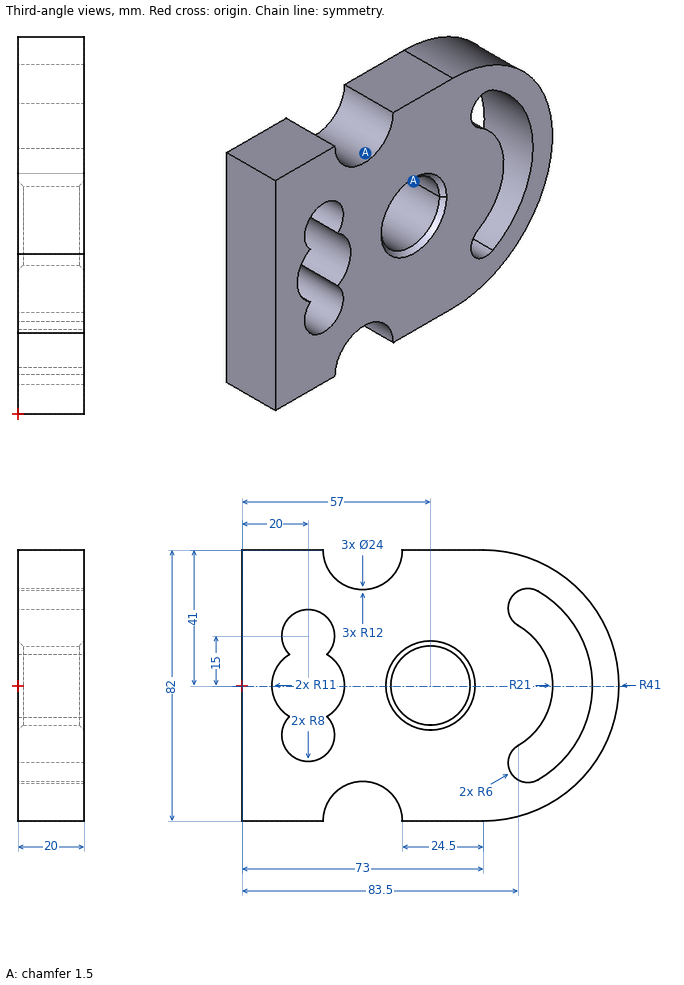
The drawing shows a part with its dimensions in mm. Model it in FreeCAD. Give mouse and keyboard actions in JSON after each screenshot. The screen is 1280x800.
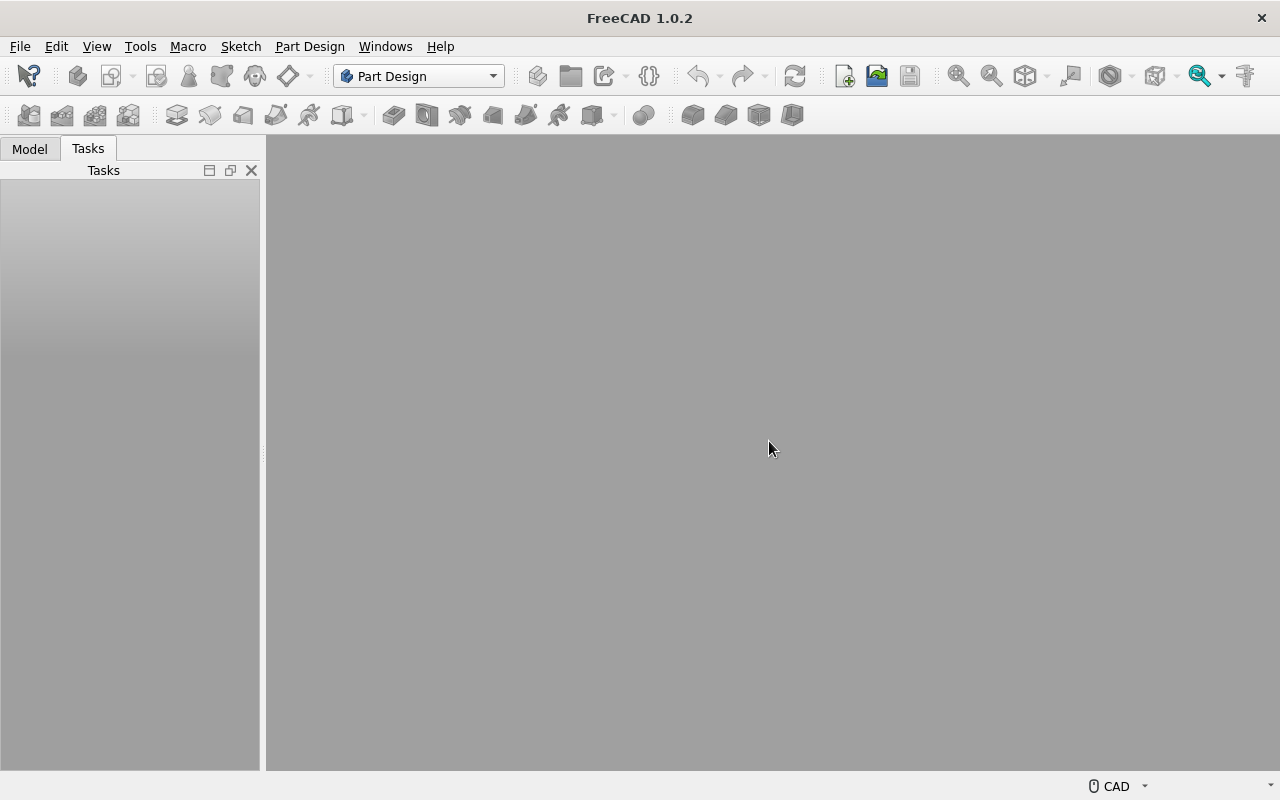
{"action": "key", "text": "ctrl+n"}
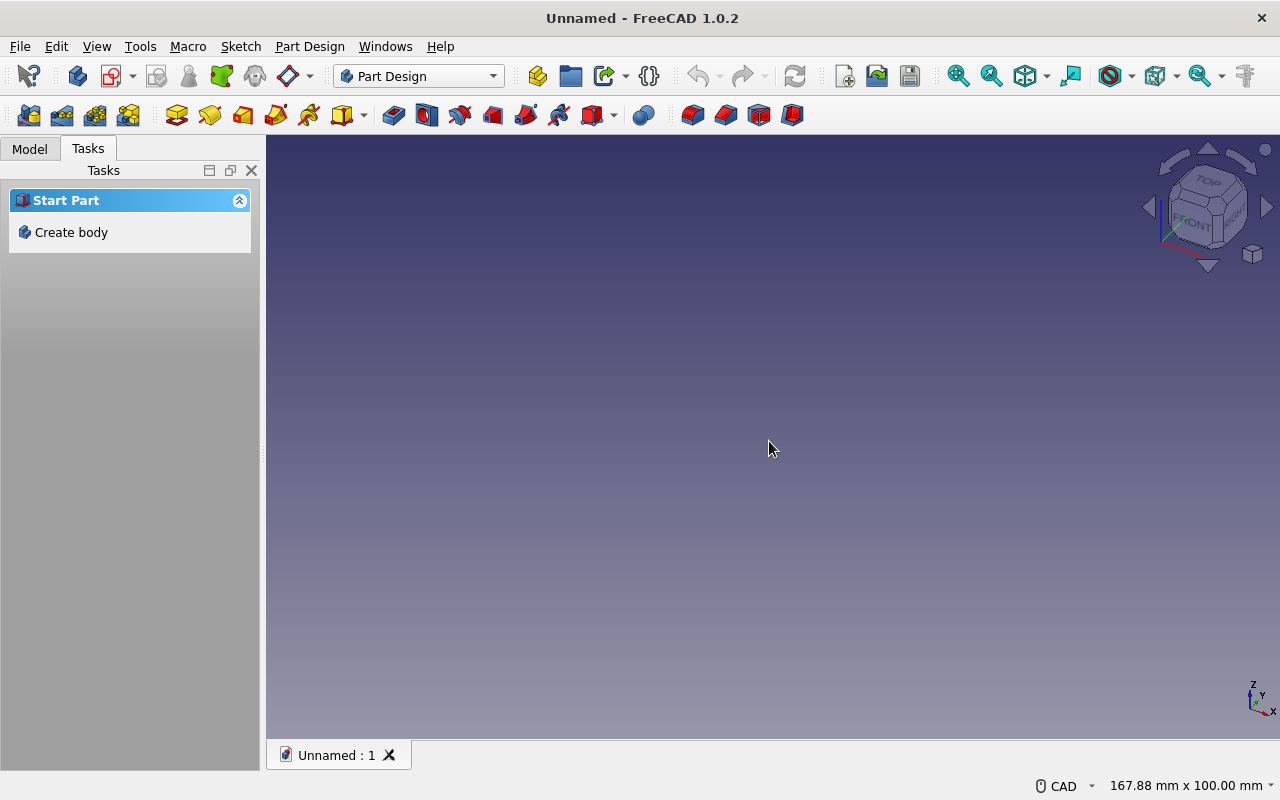
{"action": "left_click", "coordinate": [110, 76]}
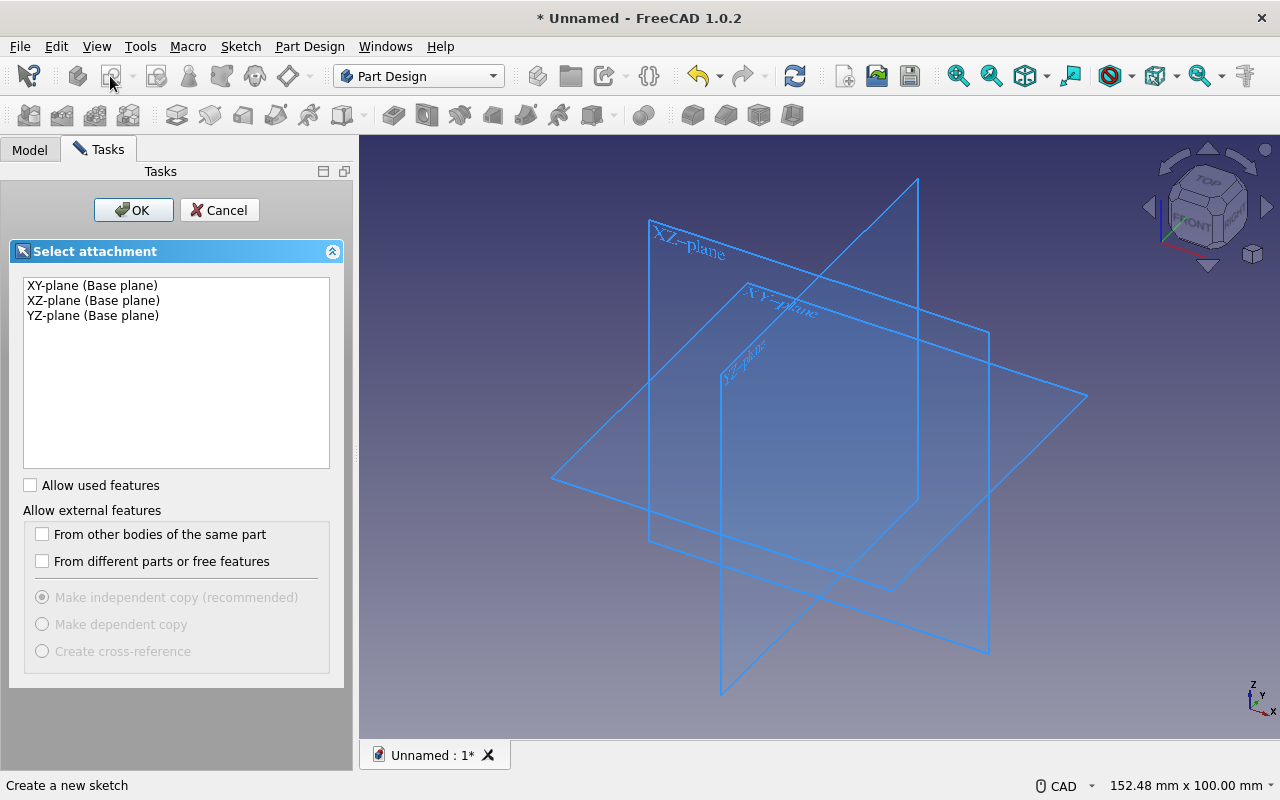
{"action": "left_click", "coordinate": [84, 316]}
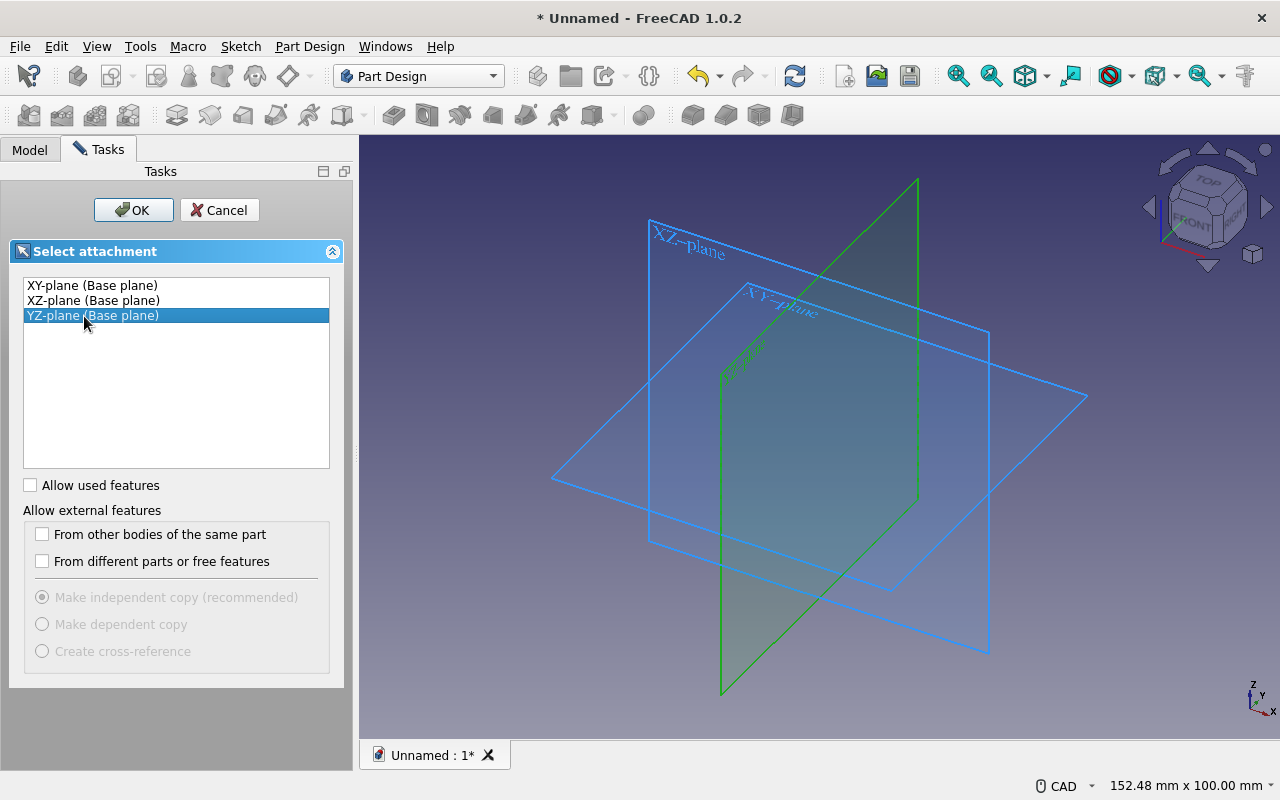
{"action": "left_click", "coordinate": [134, 210]}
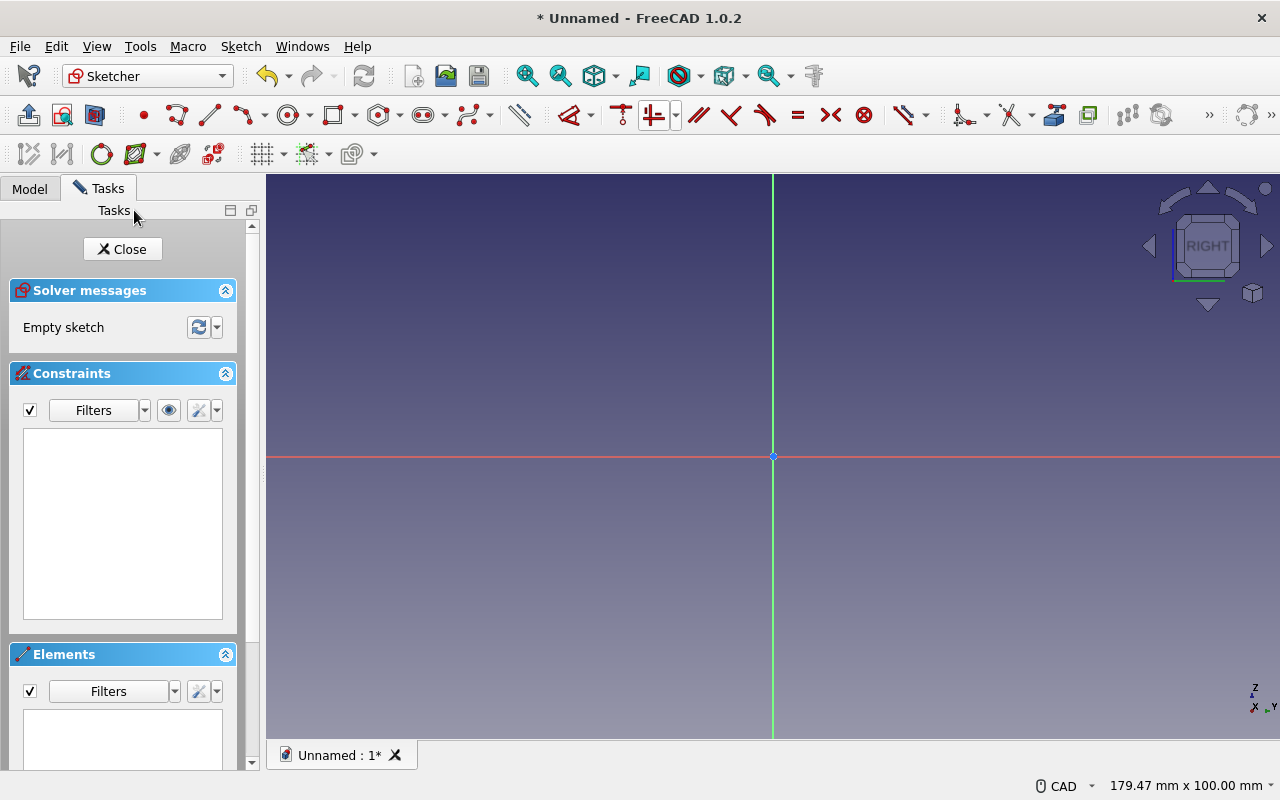
{"action": "scroll", "coordinate": [294, 457], "scroll_direction": "down", "scroll_amount": 2}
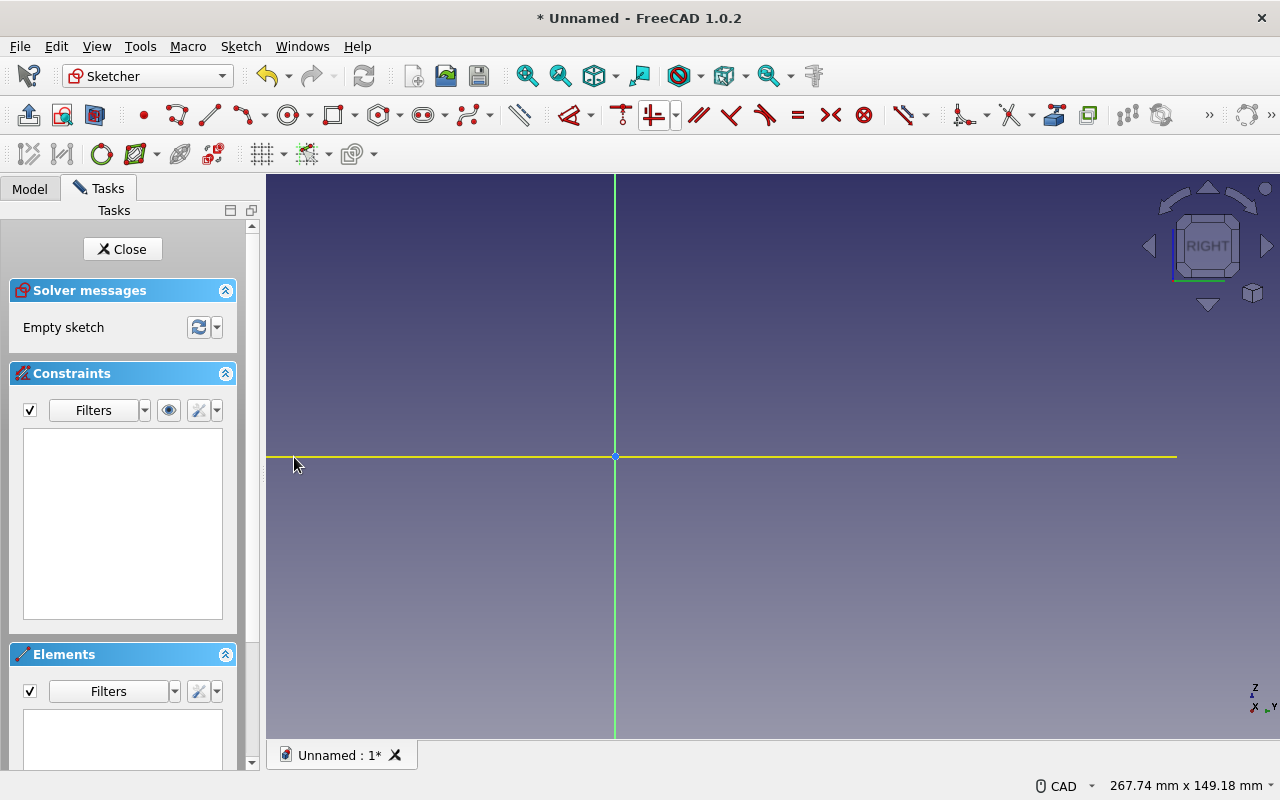
{"action": "left_click", "coordinate": [210, 116]}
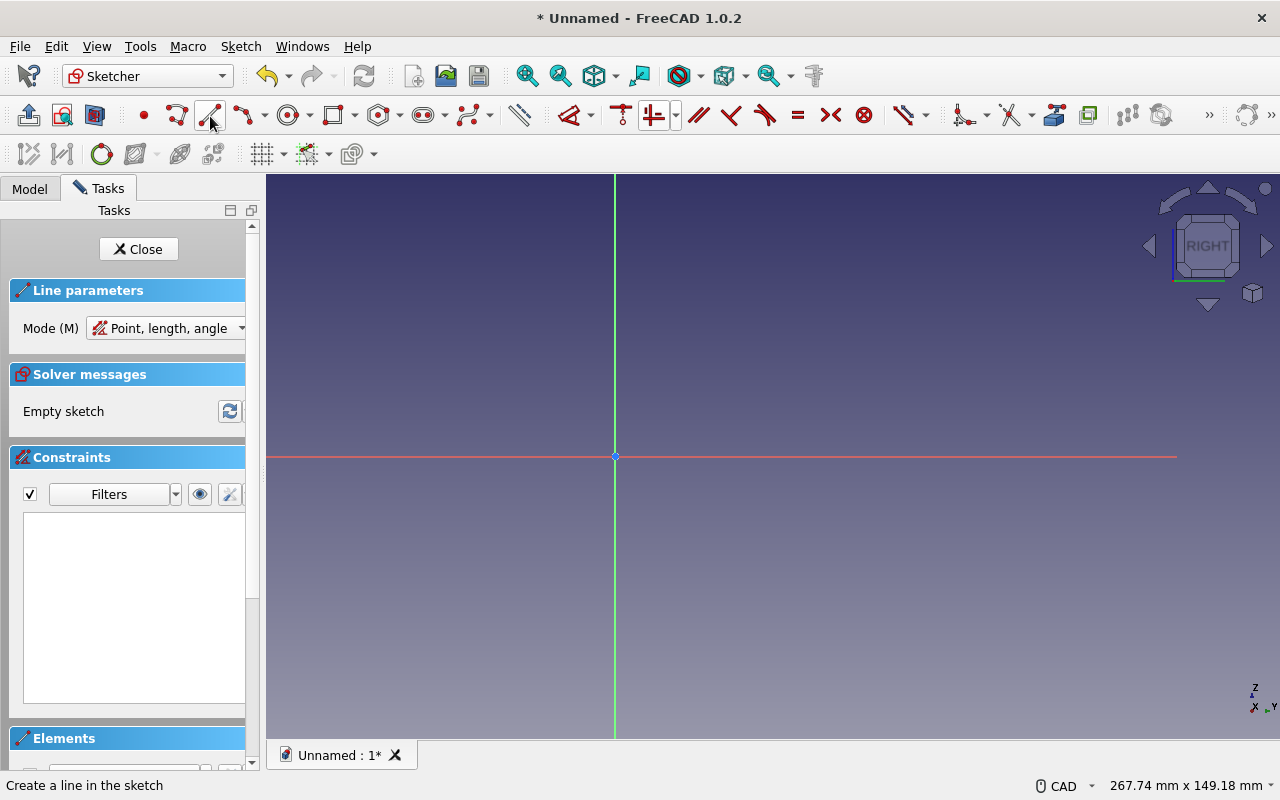
{"action": "left_click", "coordinate": [799, 612]}
{"action": "left_click", "coordinate": [892, 612]}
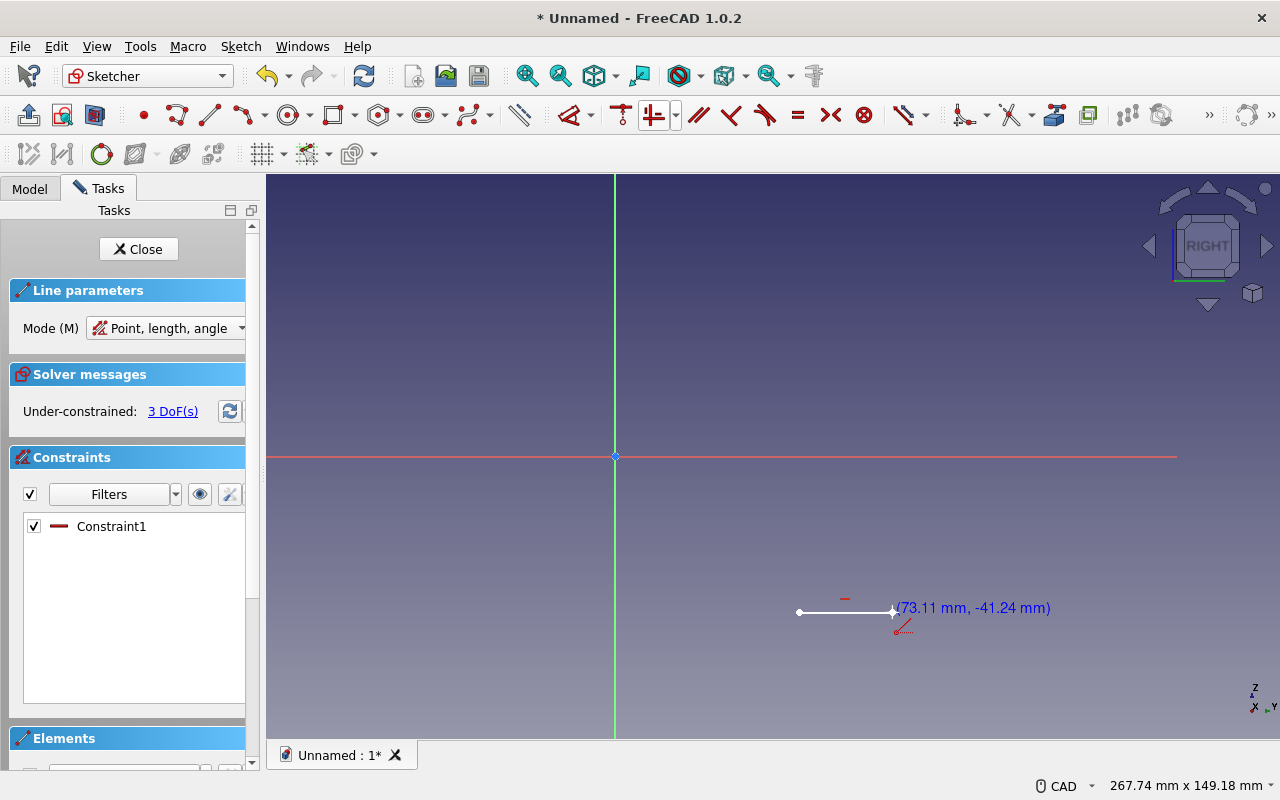
{"action": "left_click", "coordinate": [892, 302]}
{"action": "left_click", "coordinate": [799, 302]}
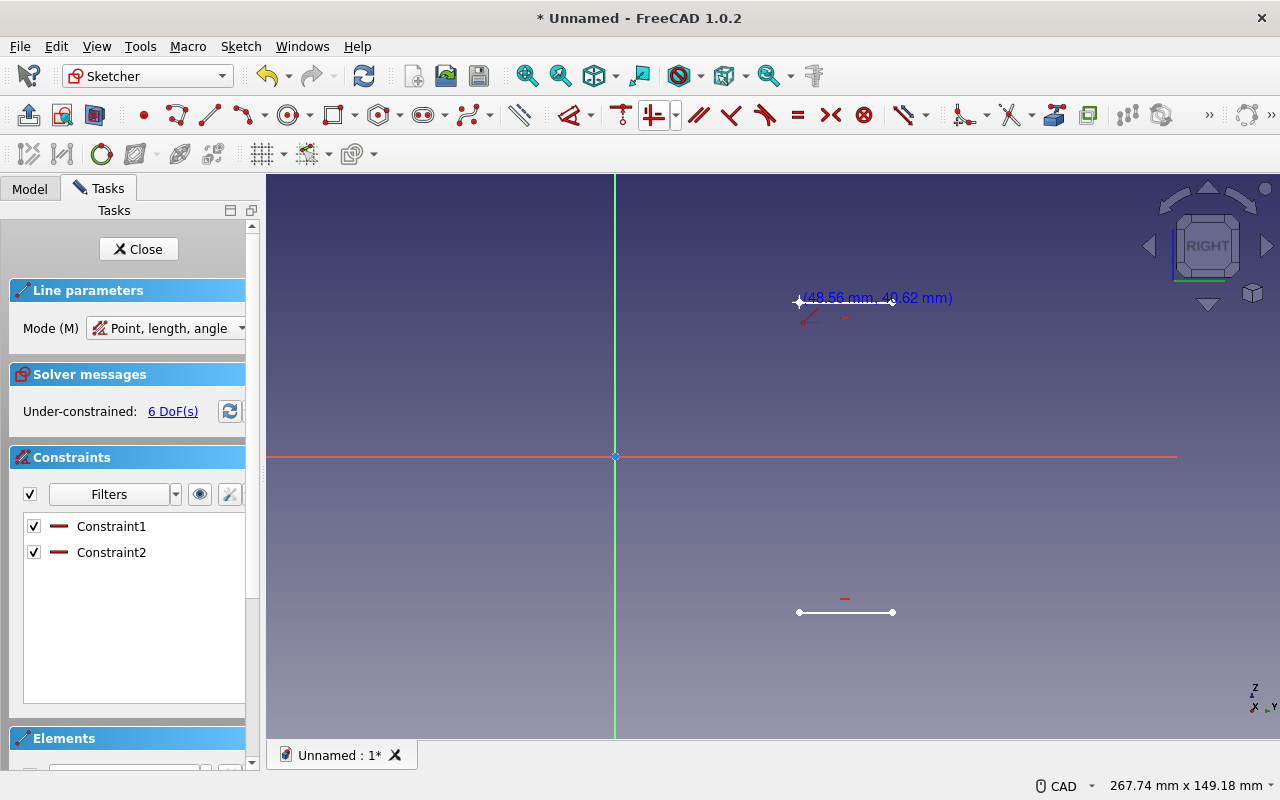
{"action": "key", "text": "g m"}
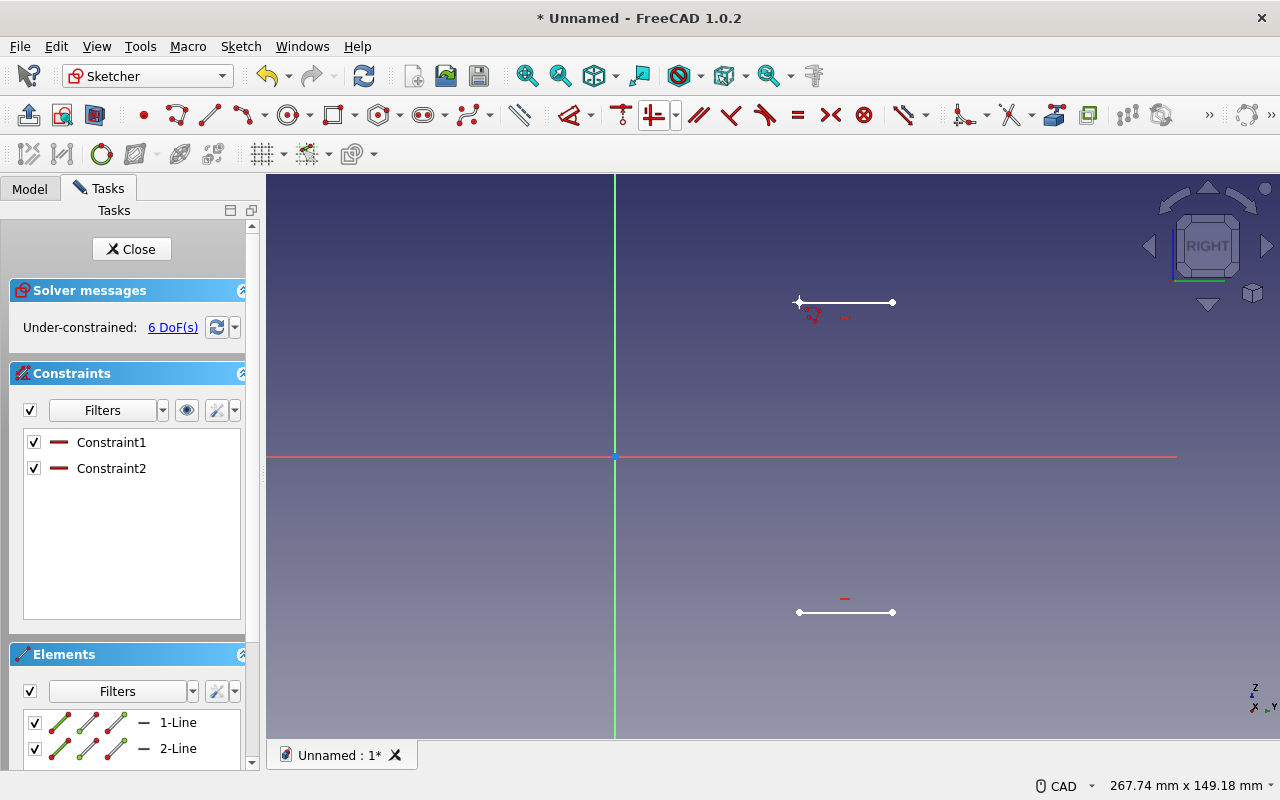
{"action": "left_click", "coordinate": [708, 302]}
{"action": "left_click", "coordinate": [615, 302]}
{"action": "left_click", "coordinate": [624, 612]}
{"action": "left_click", "coordinate": [708, 612]}
{"action": "right_click", "coordinate": [708, 612]}